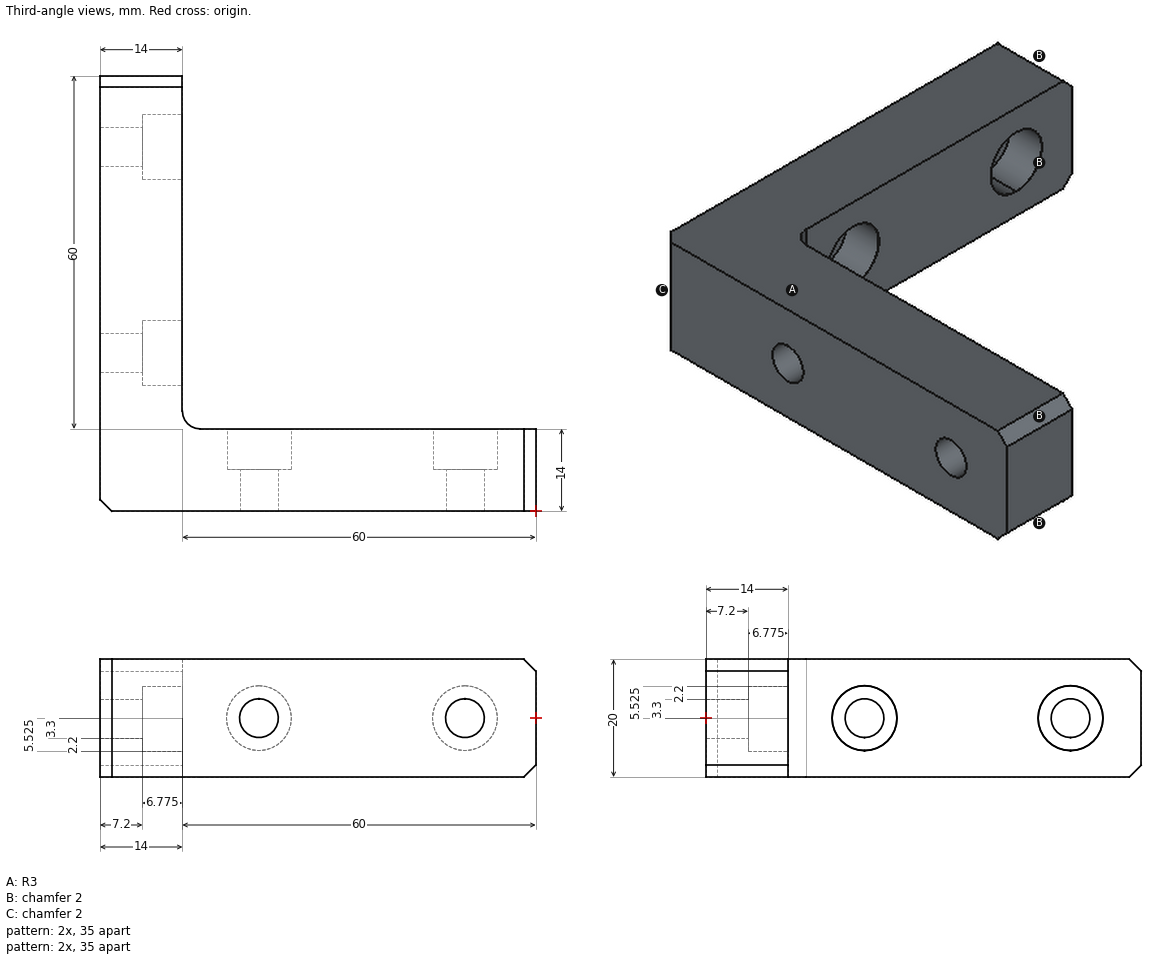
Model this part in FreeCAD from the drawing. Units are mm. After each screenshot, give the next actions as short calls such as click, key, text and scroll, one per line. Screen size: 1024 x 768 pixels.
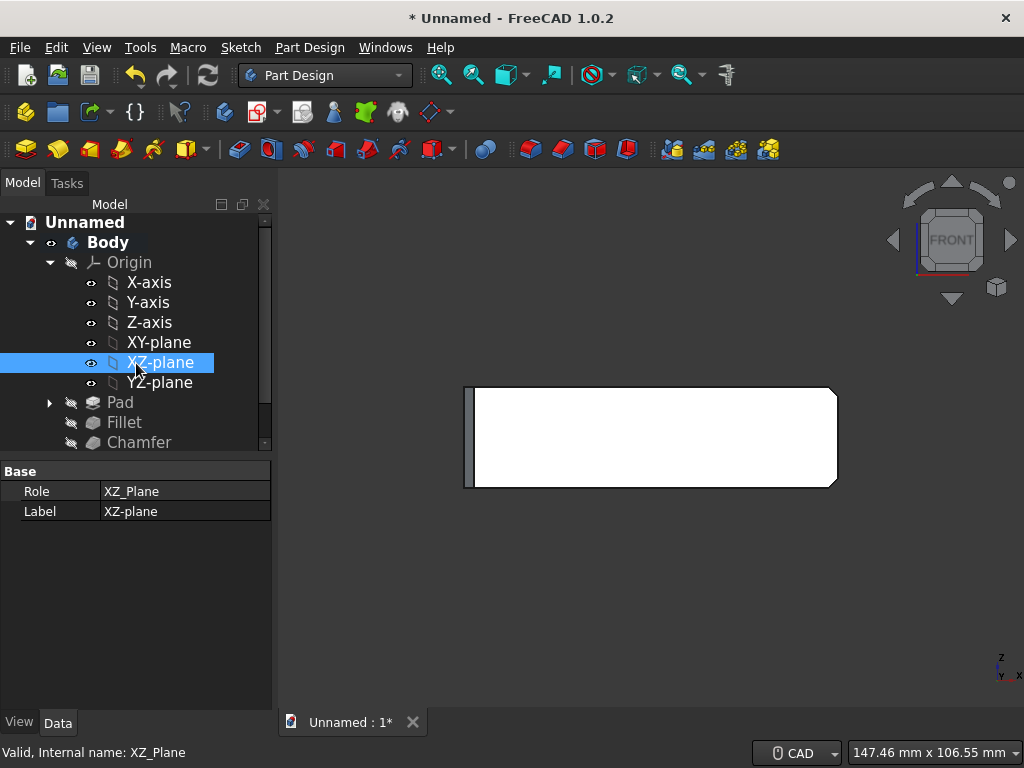
click(430, 112)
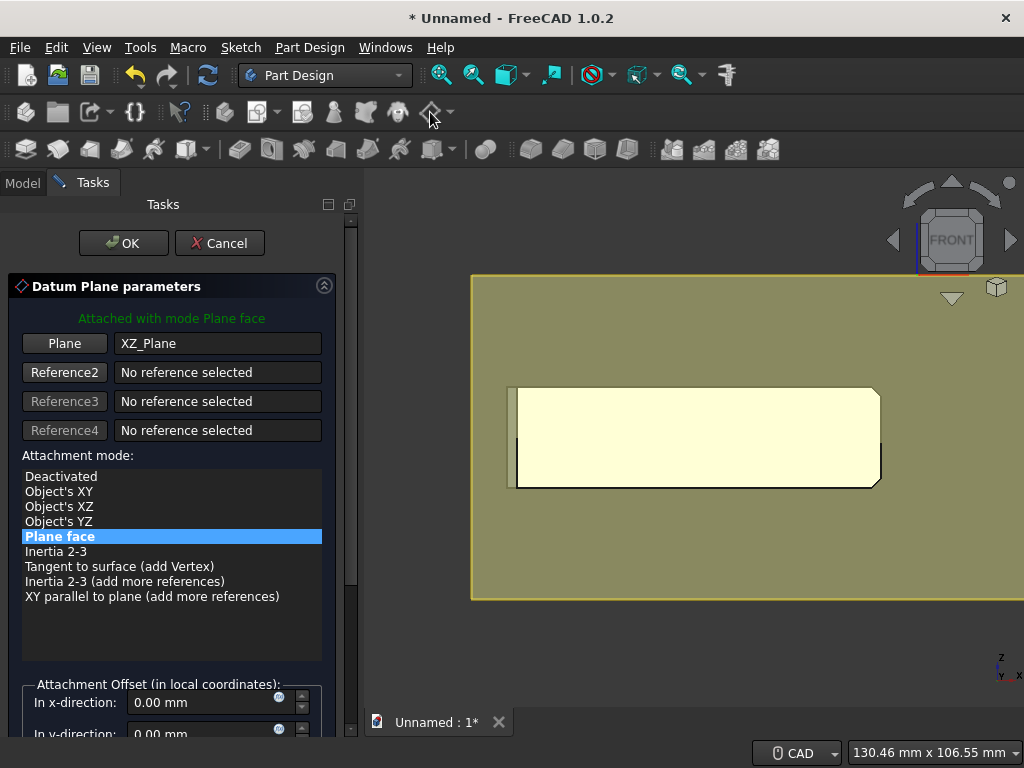
scroll(351, 475, down, 2)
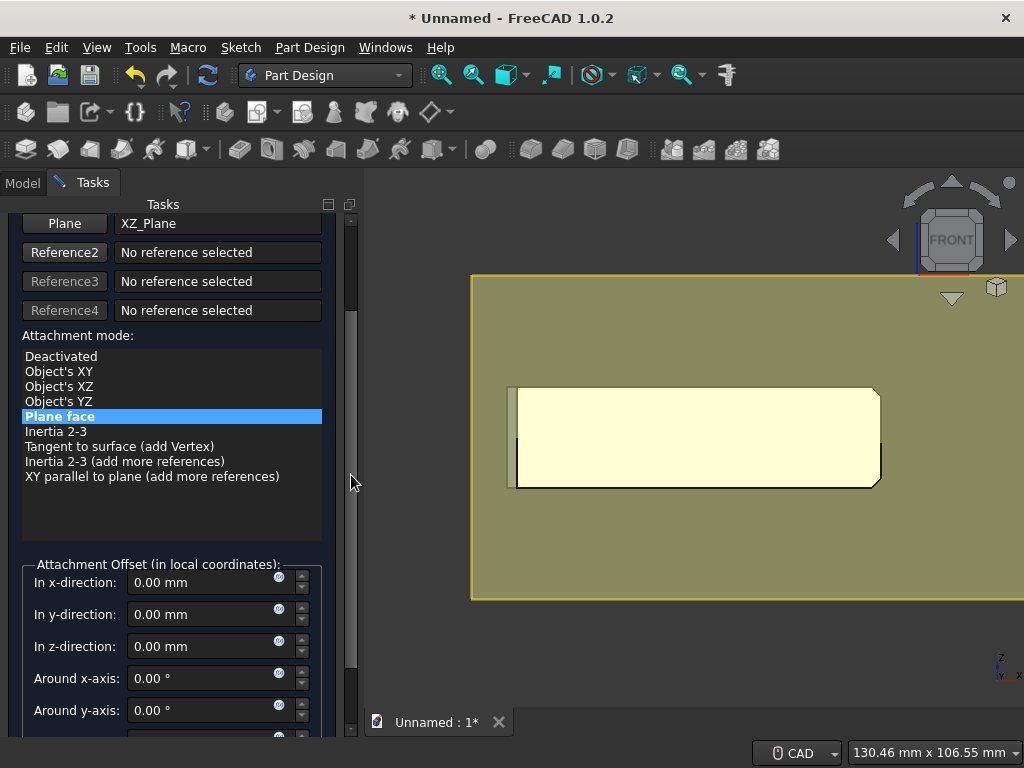
triple_click(210, 646)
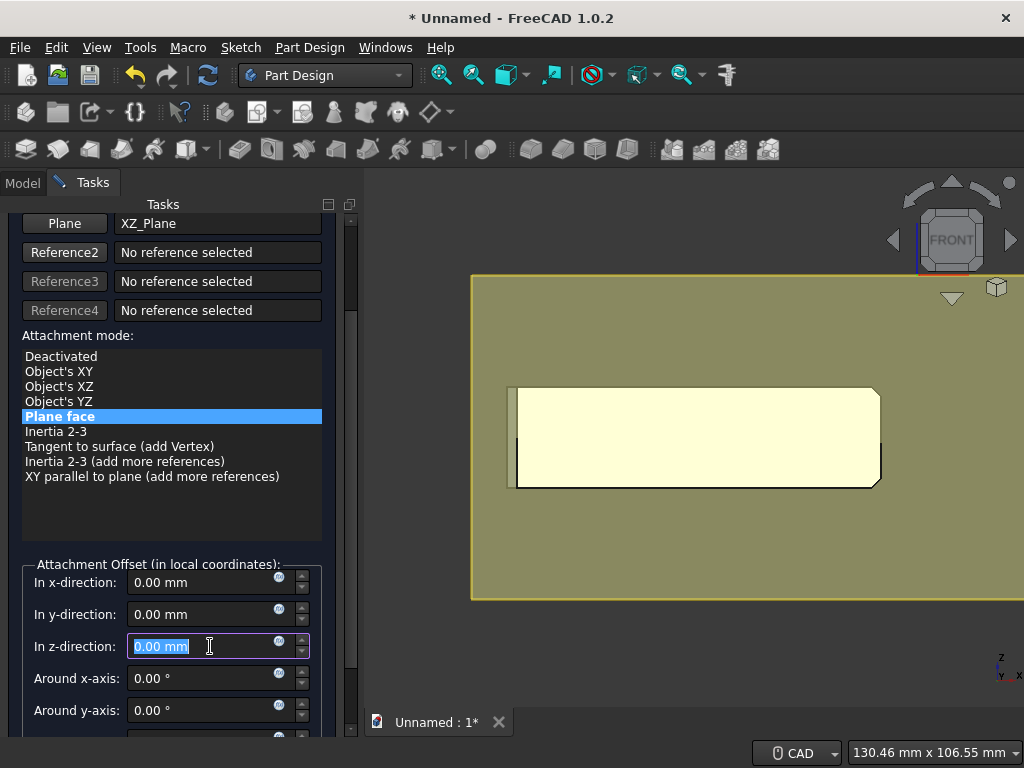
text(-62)
key(Tab)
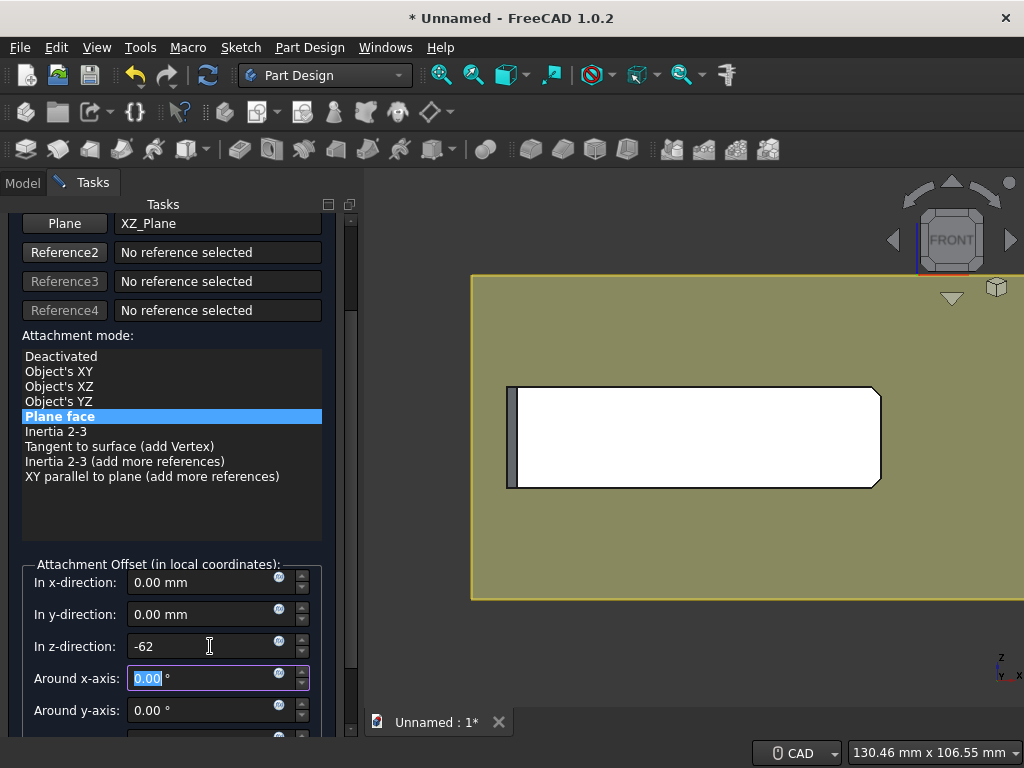
scroll(351, 475, up, 3)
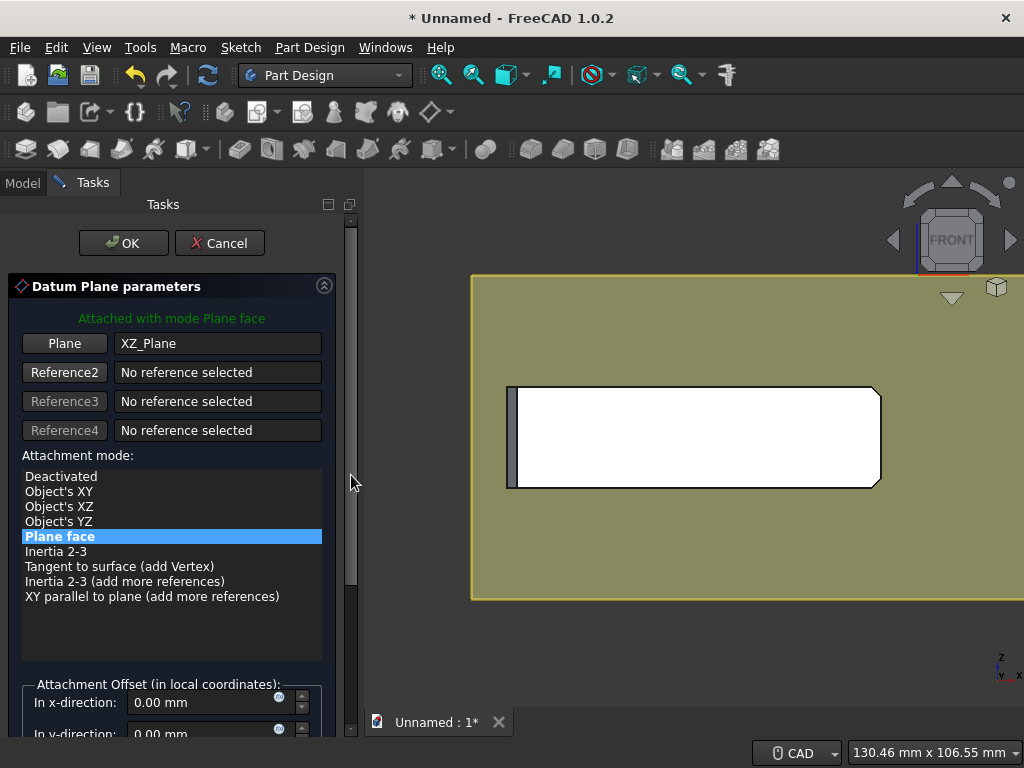
click(124, 243)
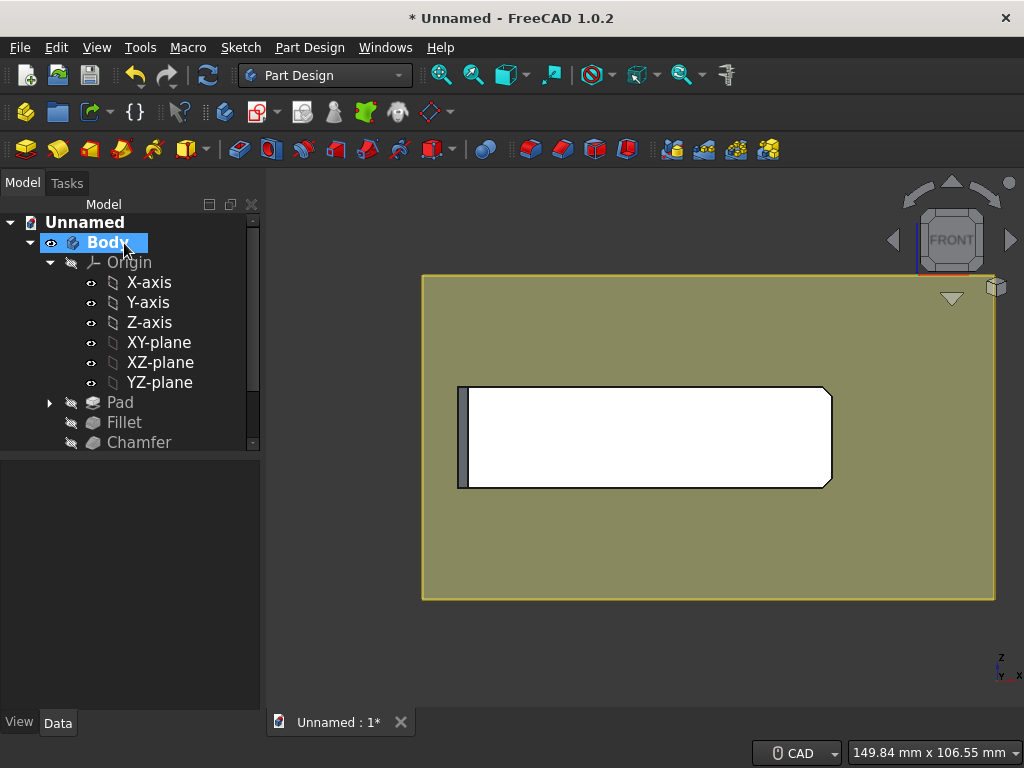
scroll(100, 338, down, 3)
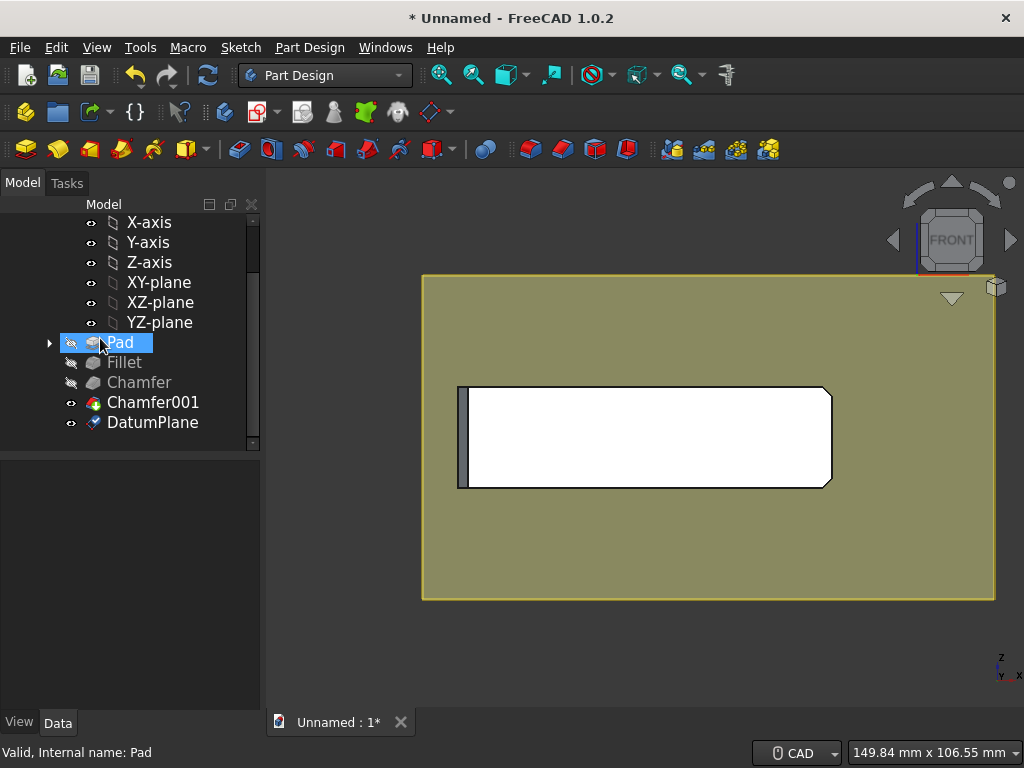
click(116, 423)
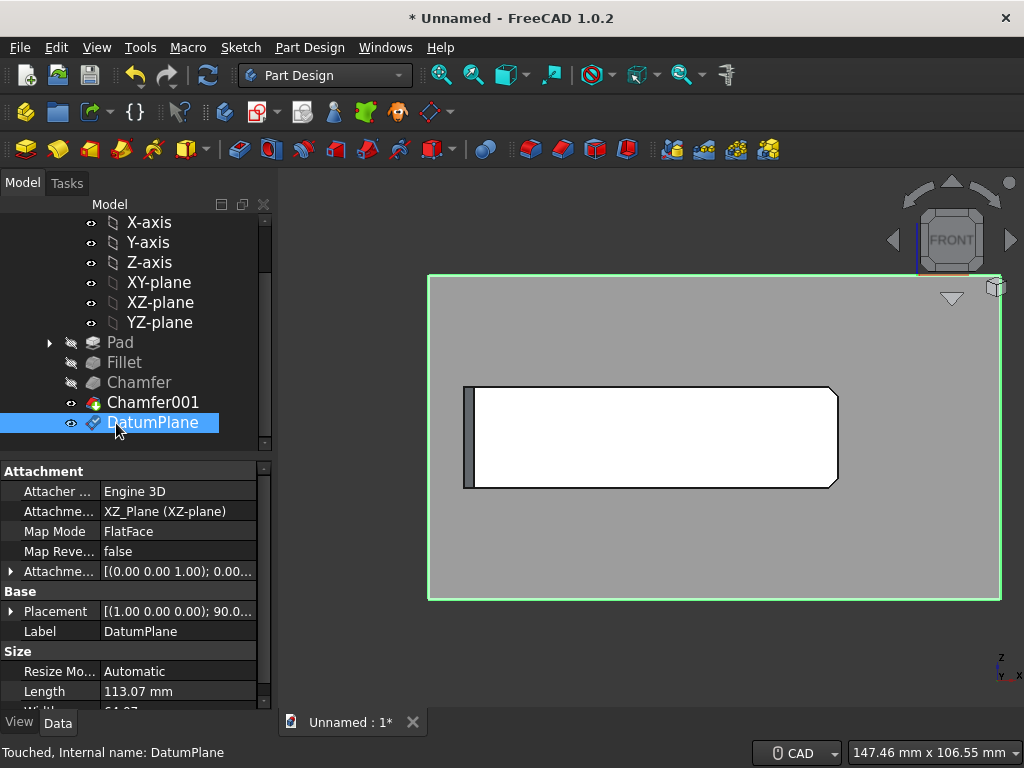
click(258, 112)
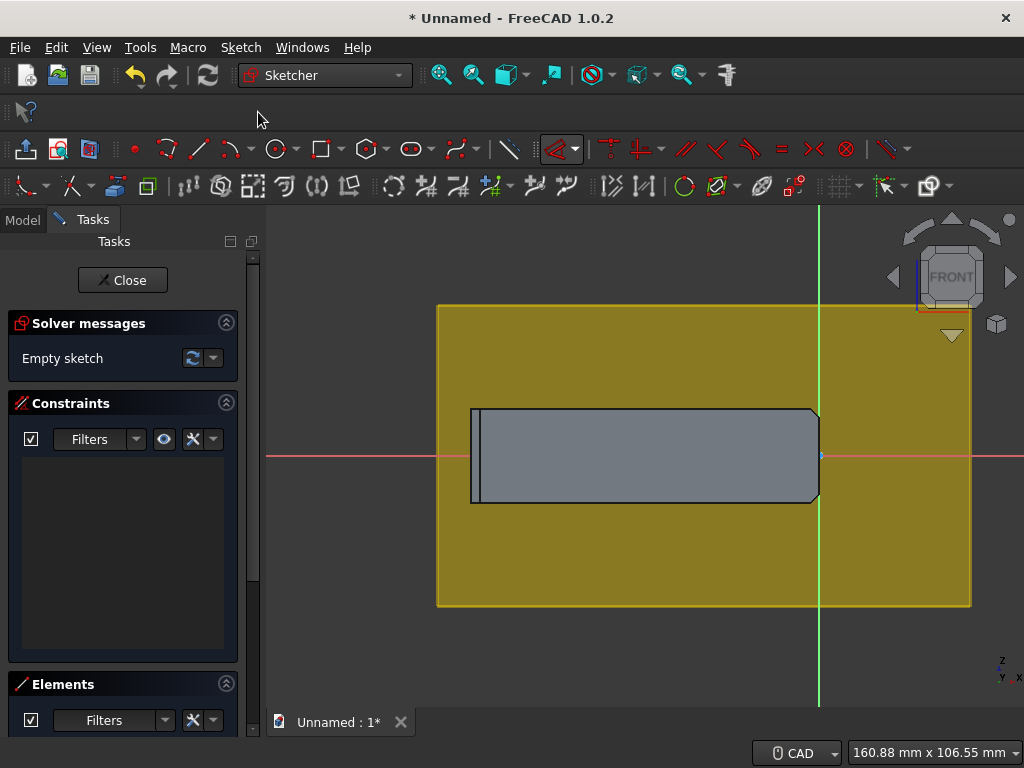
click(90, 150)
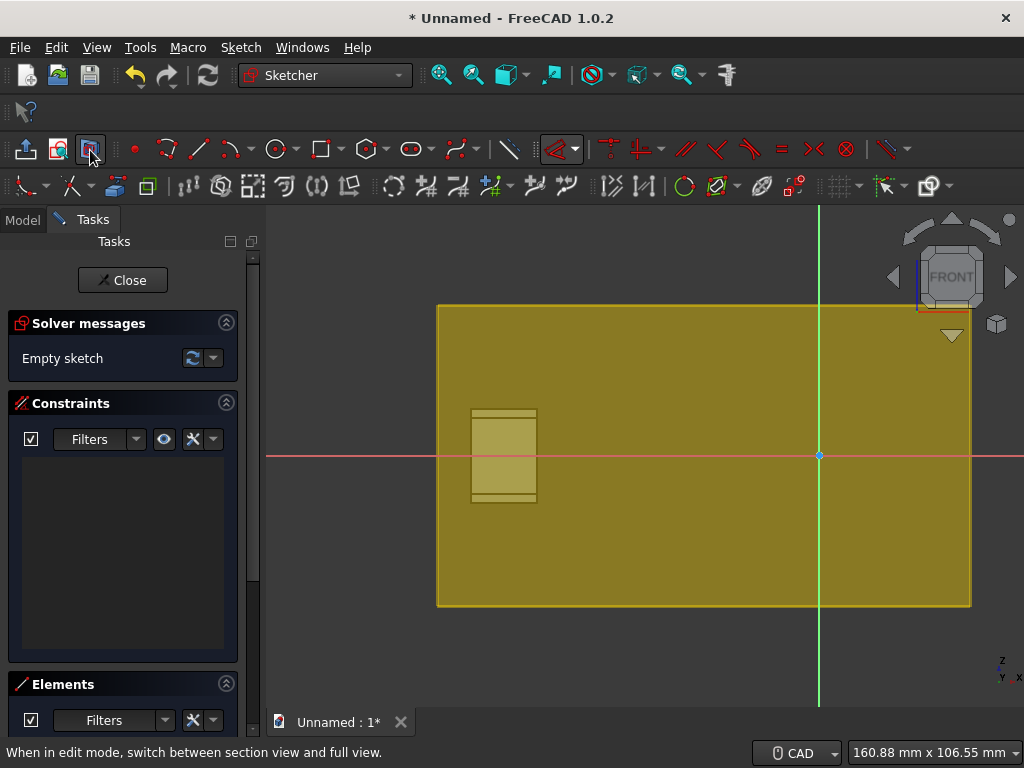
scroll(489, 472, up, 9)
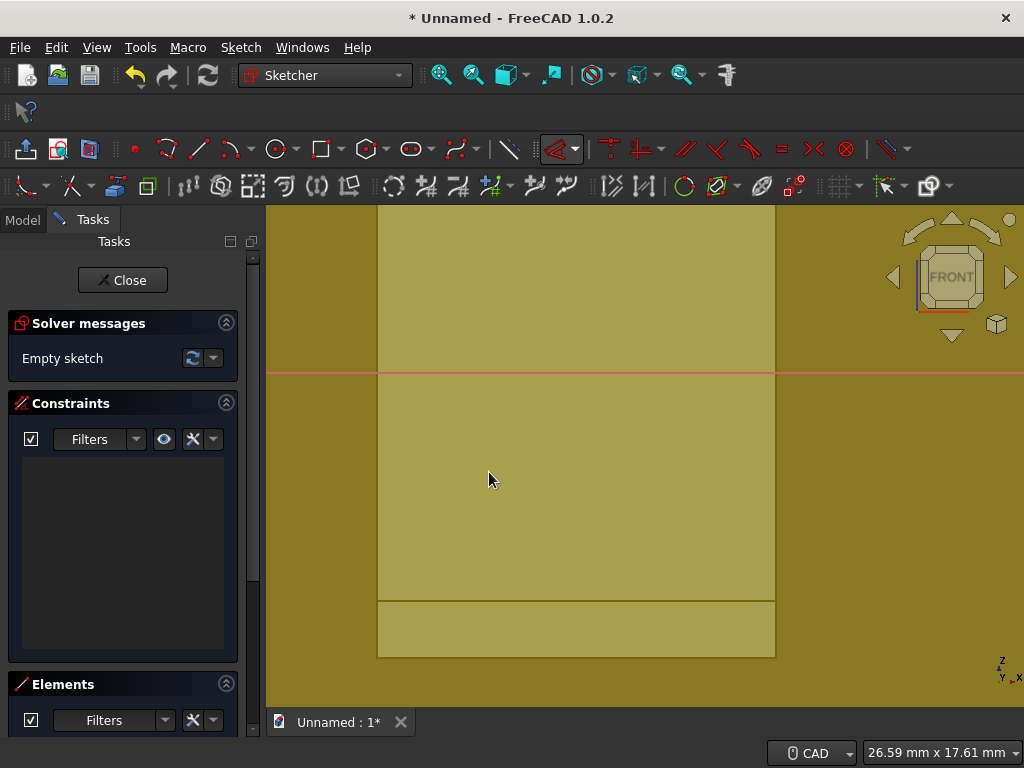
click(168, 150)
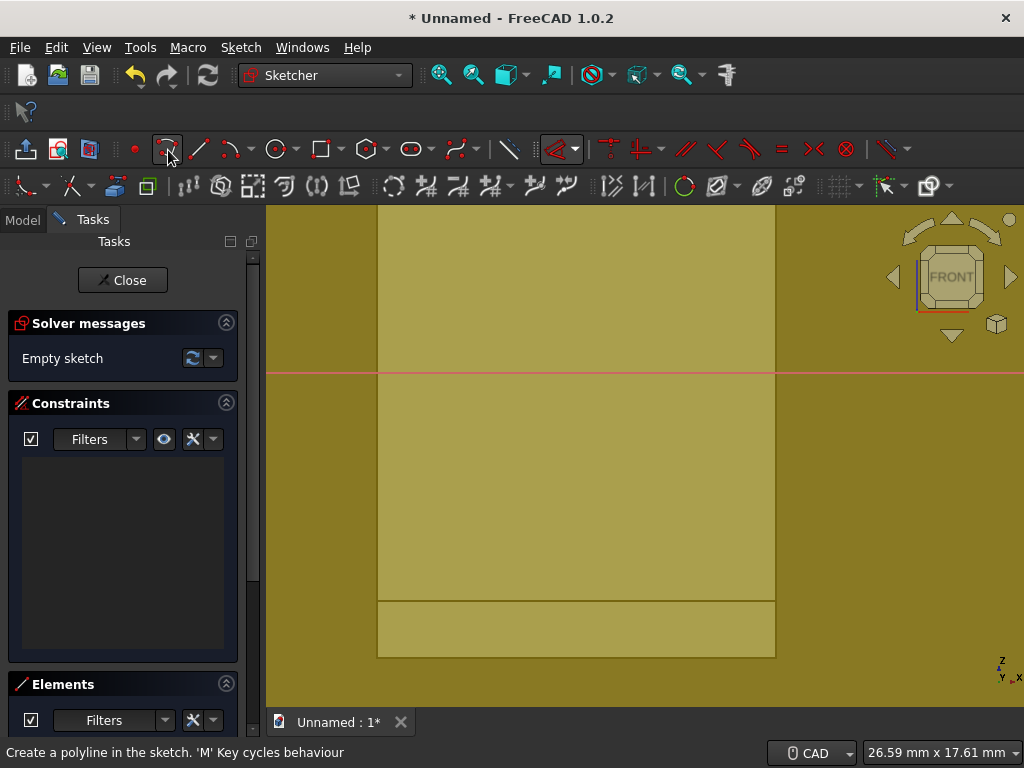
click(776, 373)
click(776, 530)